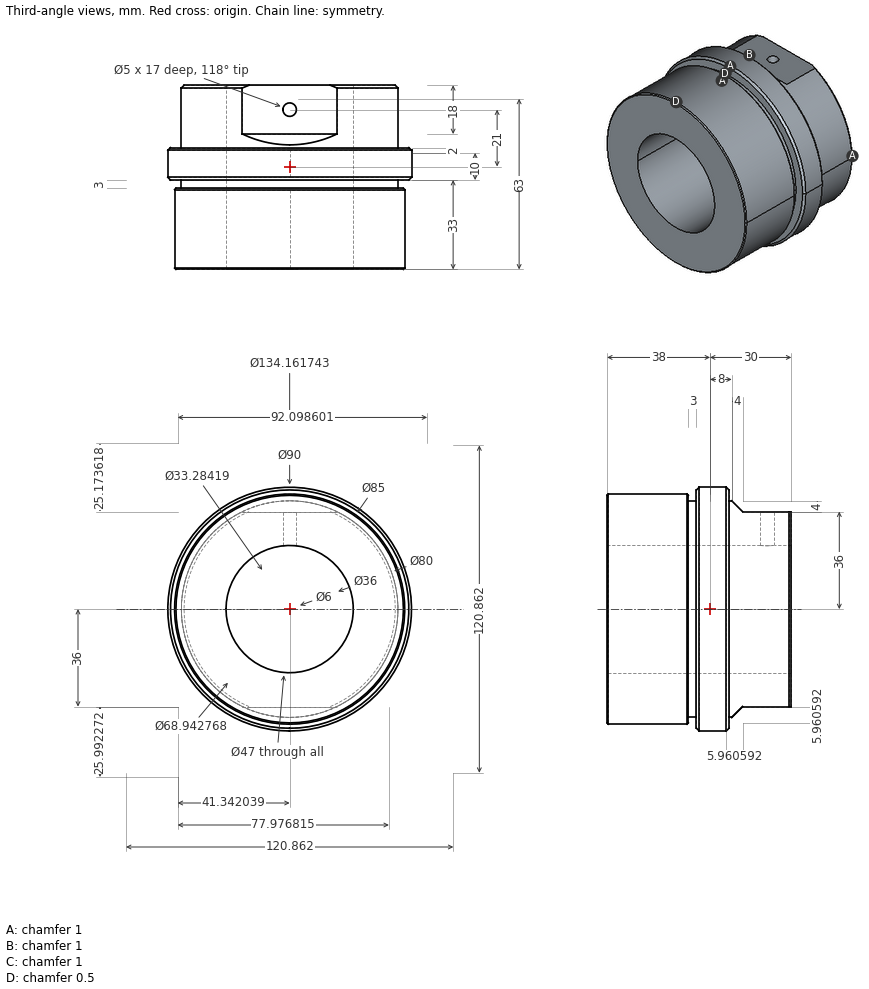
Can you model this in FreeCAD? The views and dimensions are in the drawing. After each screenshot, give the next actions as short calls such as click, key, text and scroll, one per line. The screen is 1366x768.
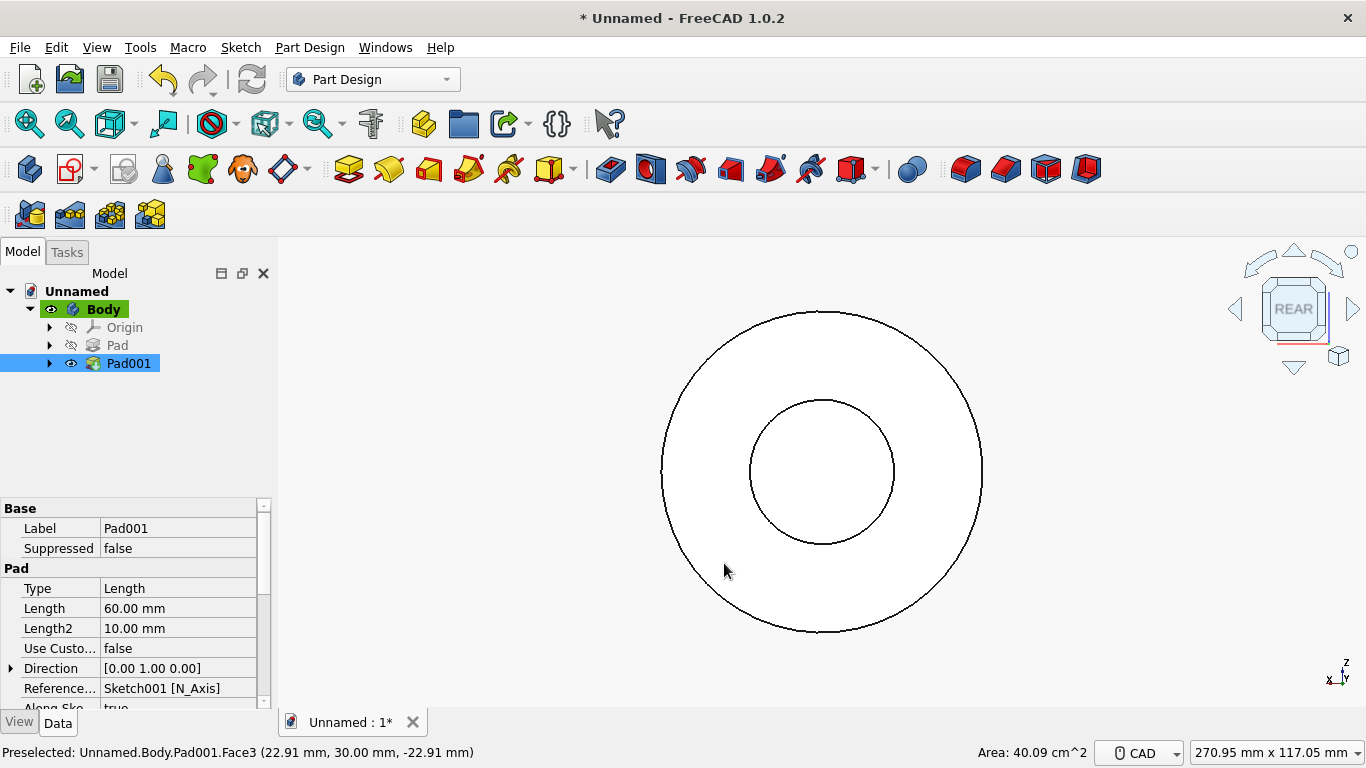
click(70, 170)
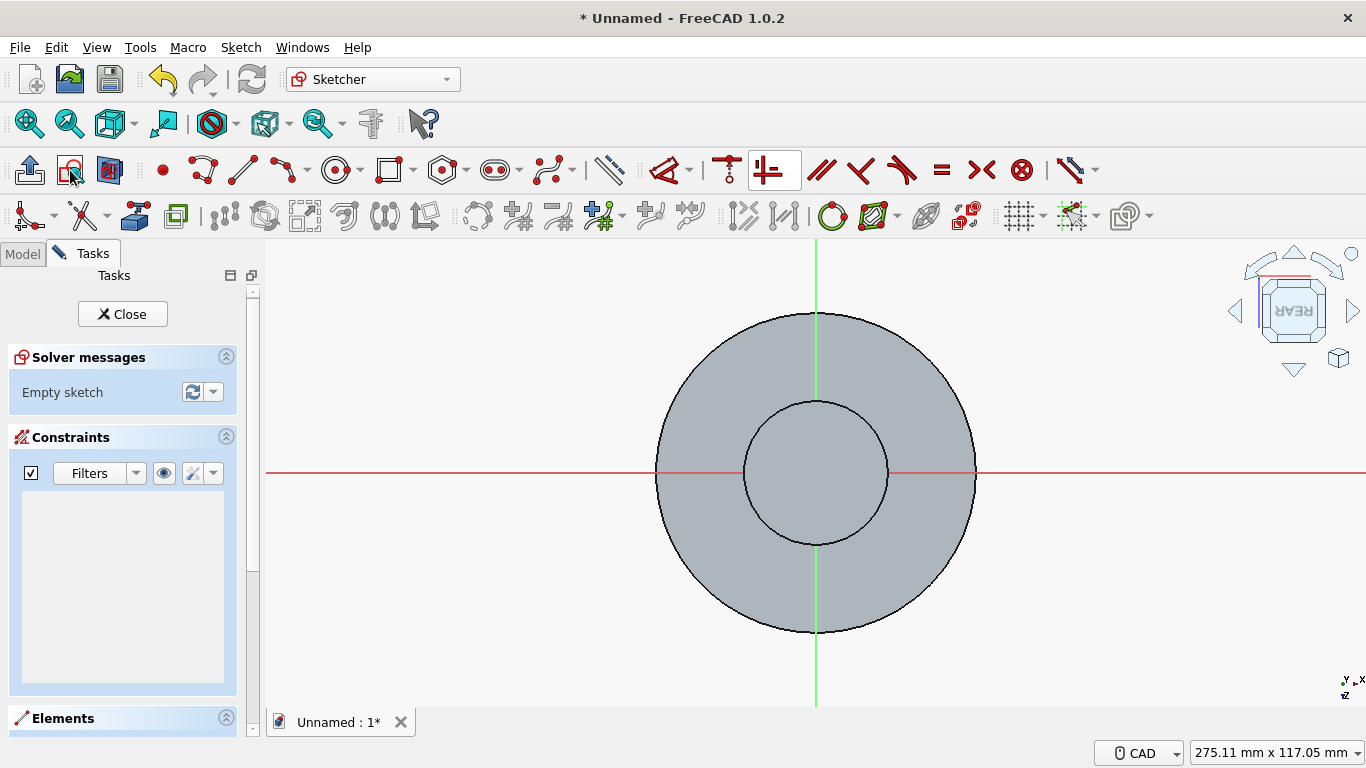
scroll(641, 475, down, 3)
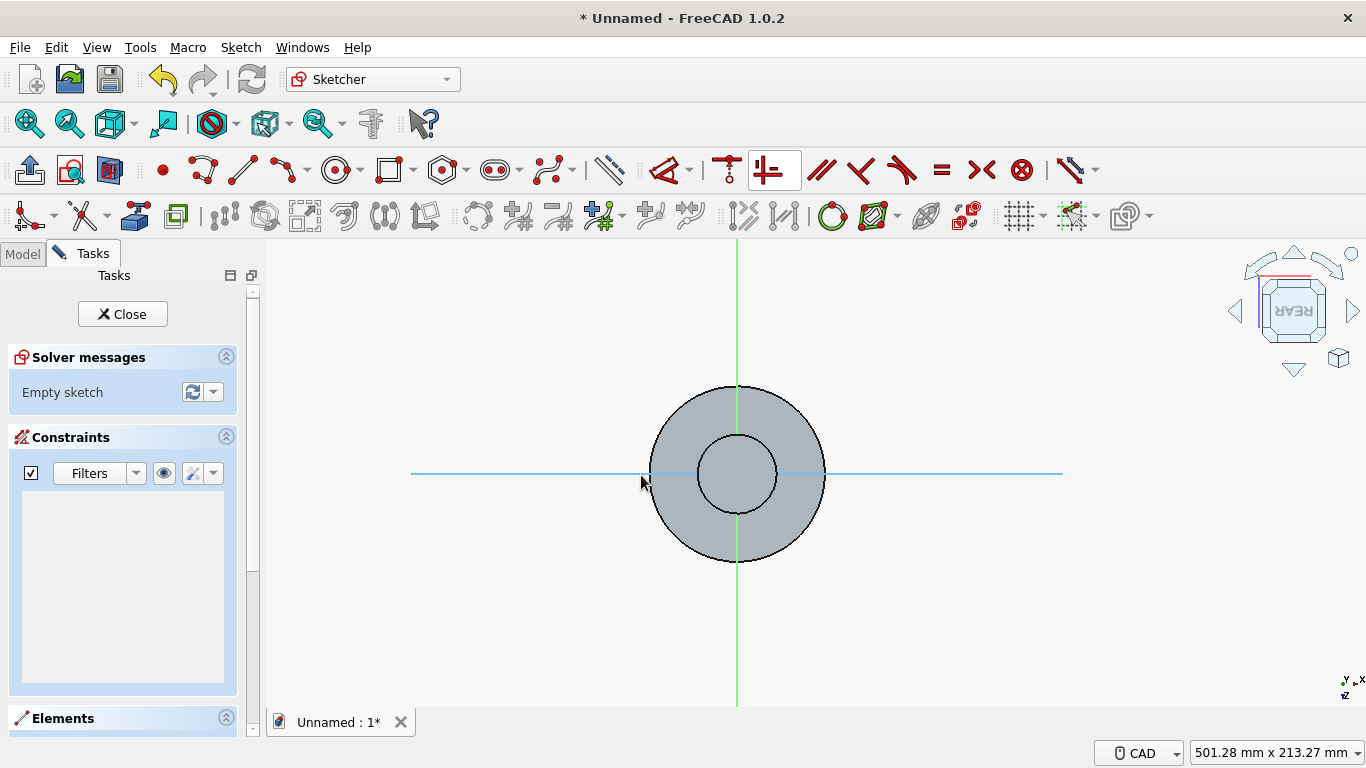
click(390, 170)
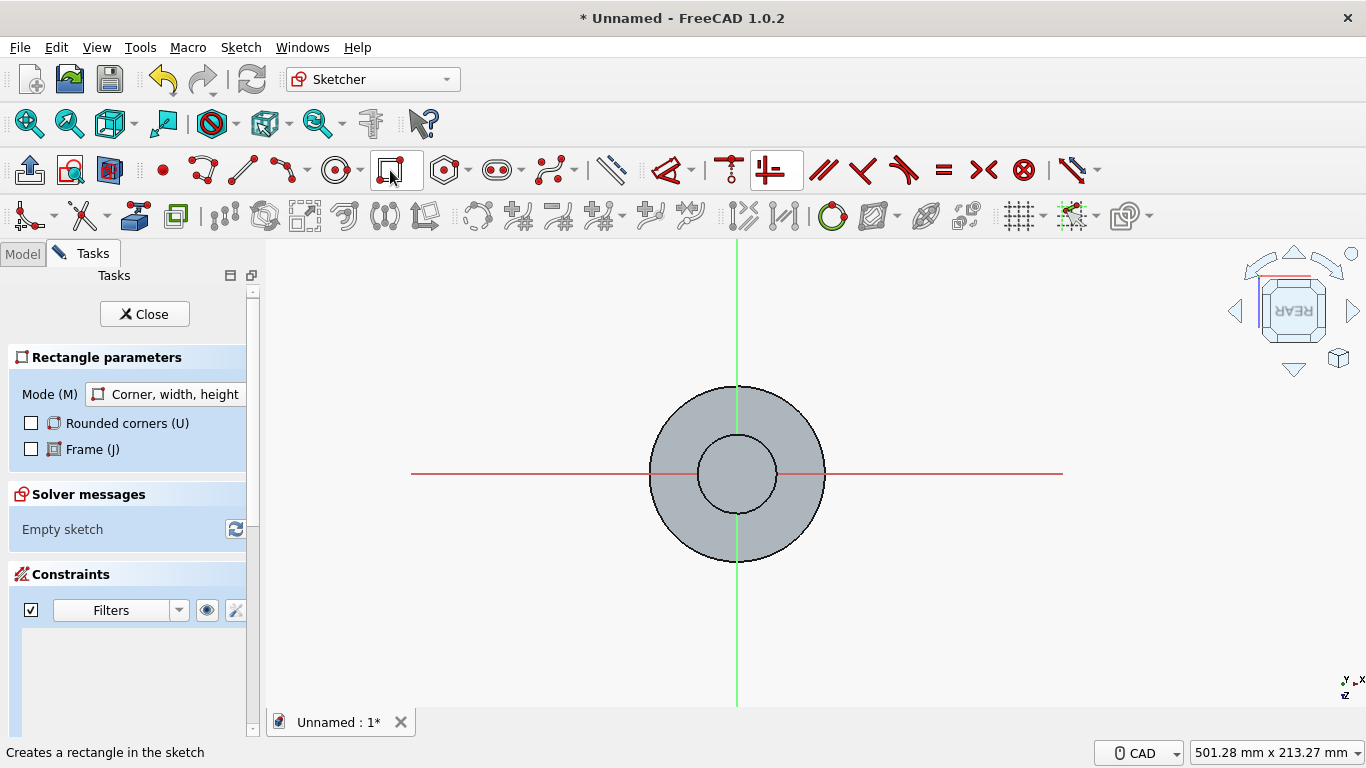
click(646, 338)
click(818, 395)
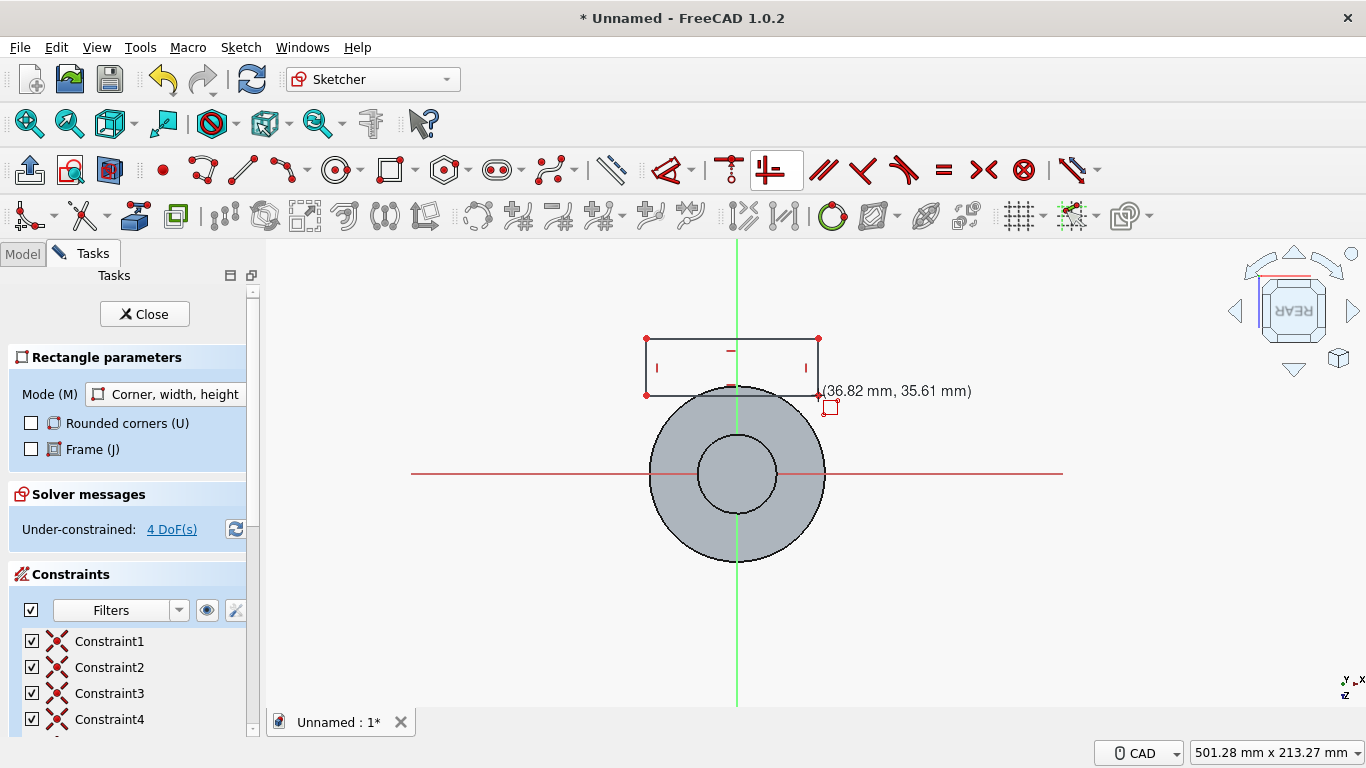
click(646, 553)
click(849, 608)
key(Escape)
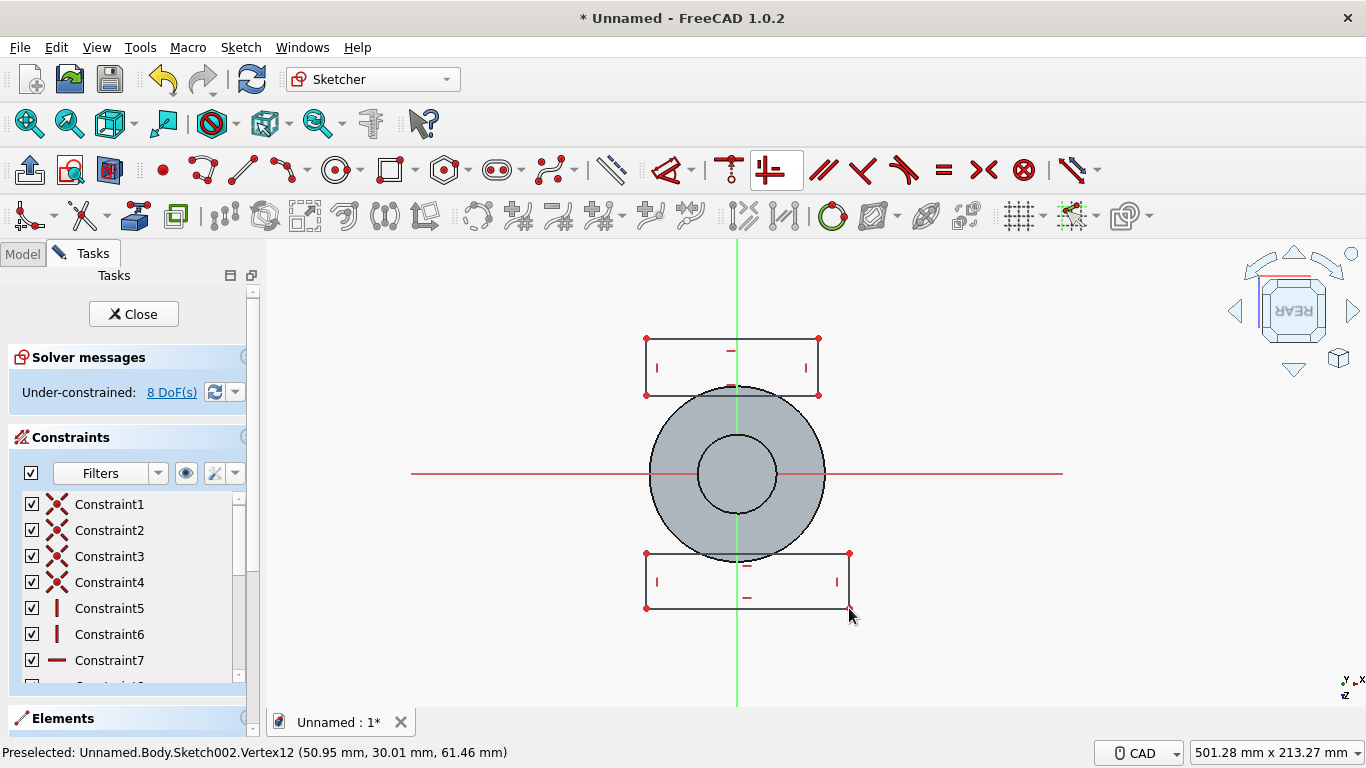
click(646, 396)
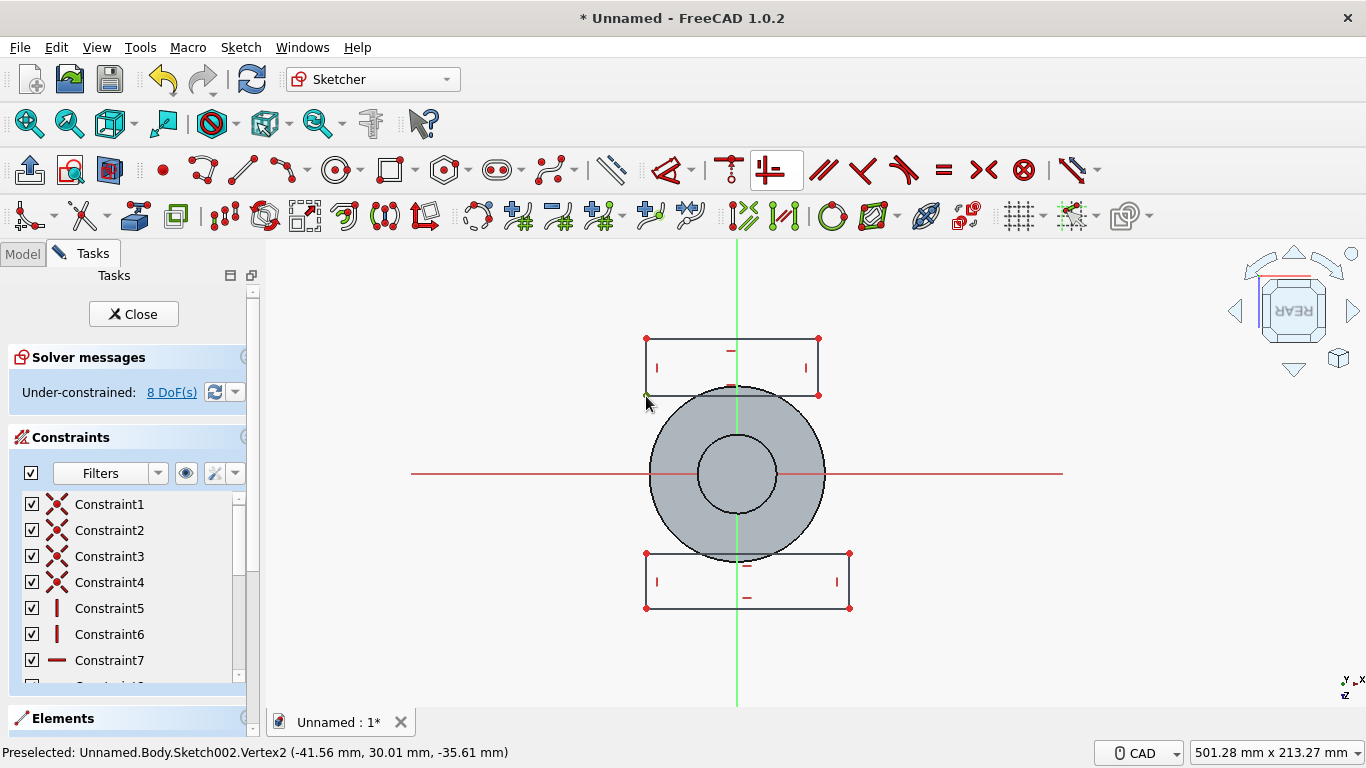
click(646, 554)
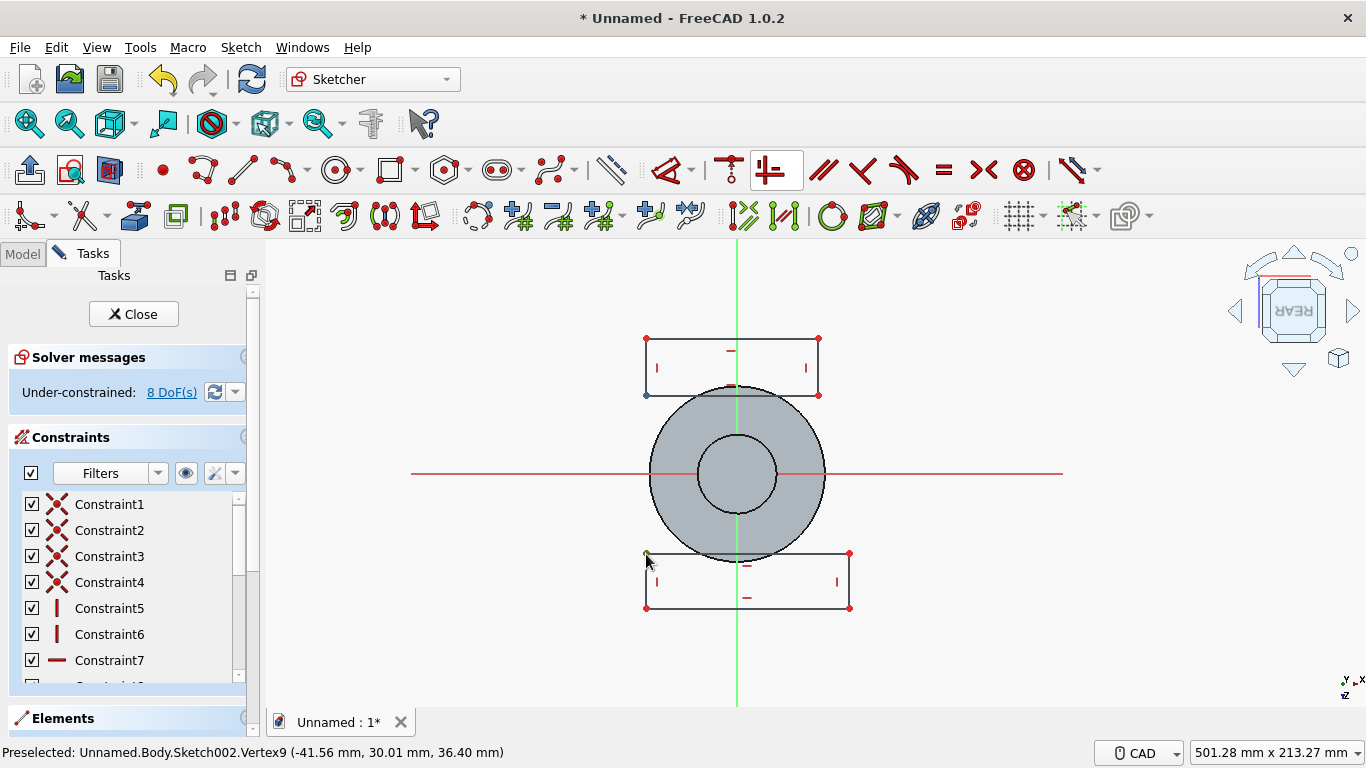
click(424, 474)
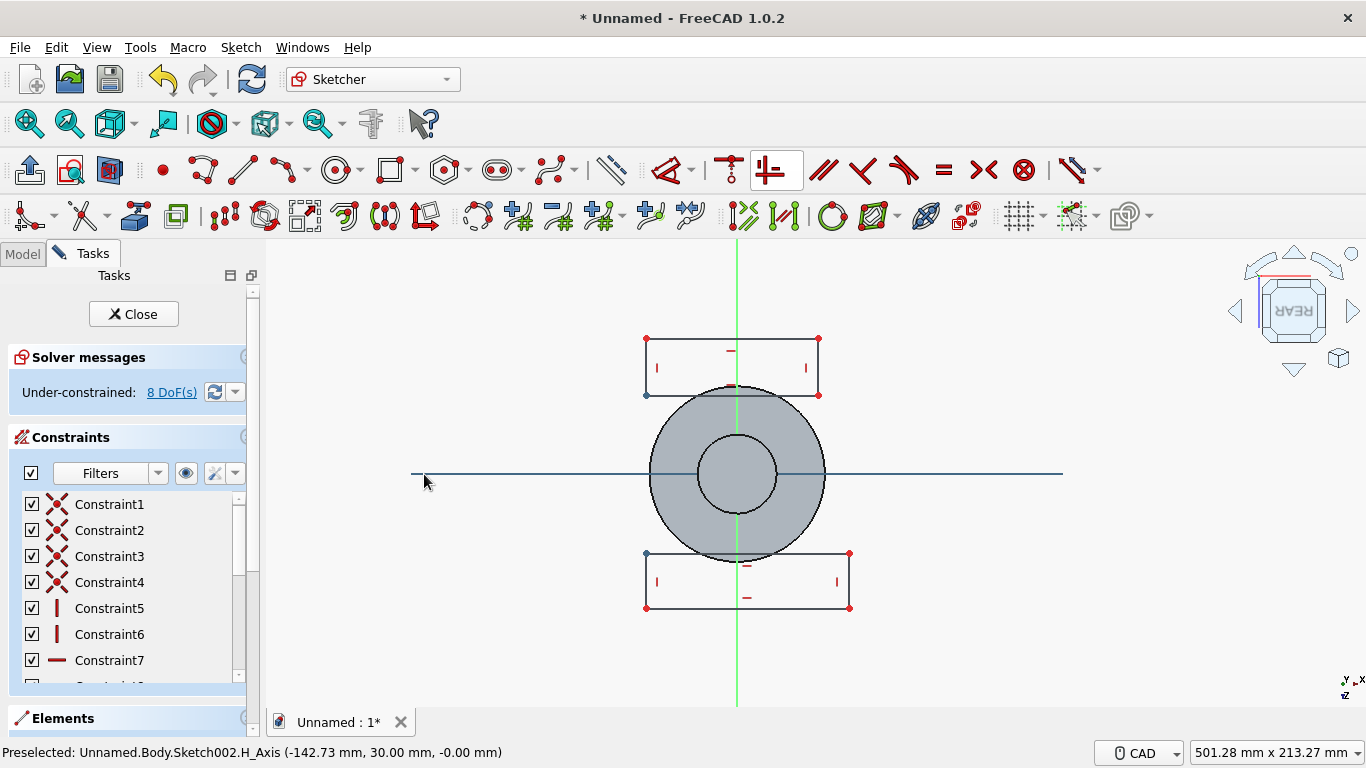
click(984, 170)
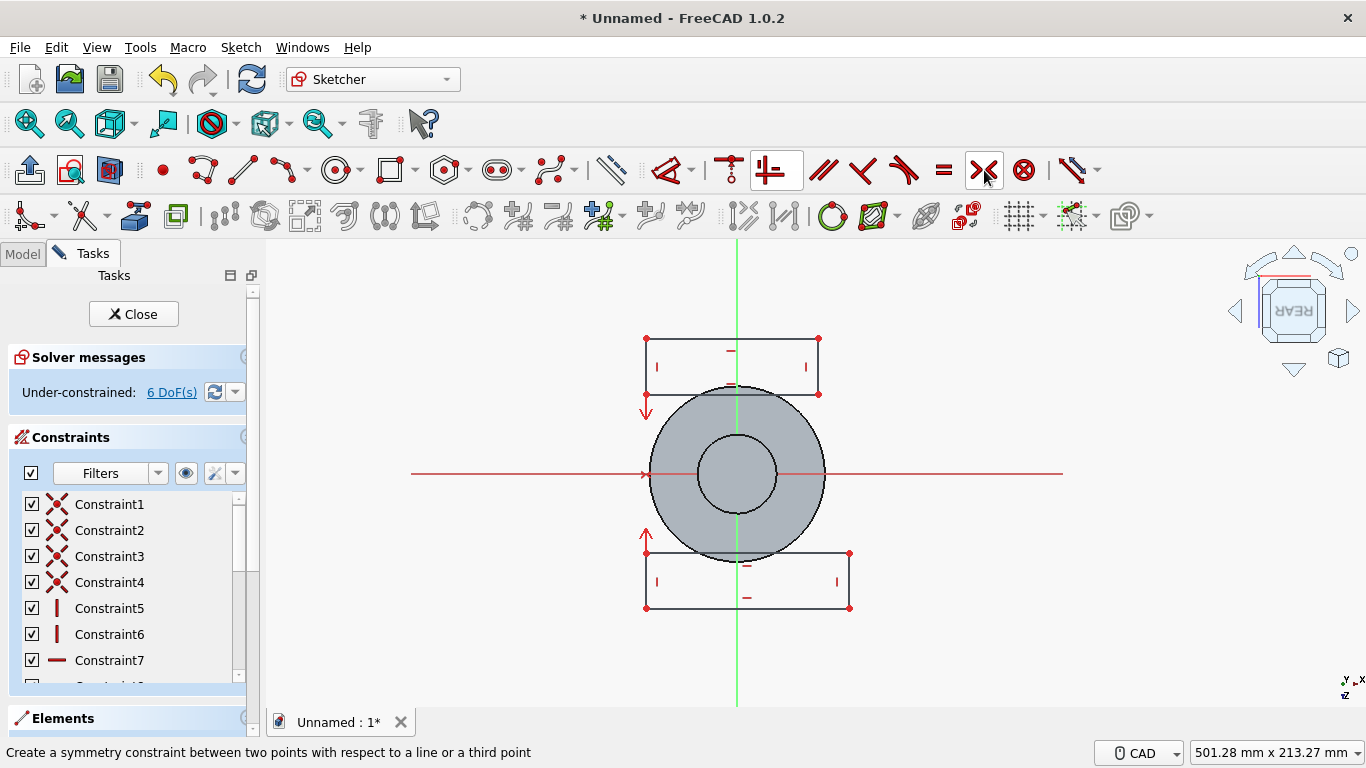
click(666, 170)